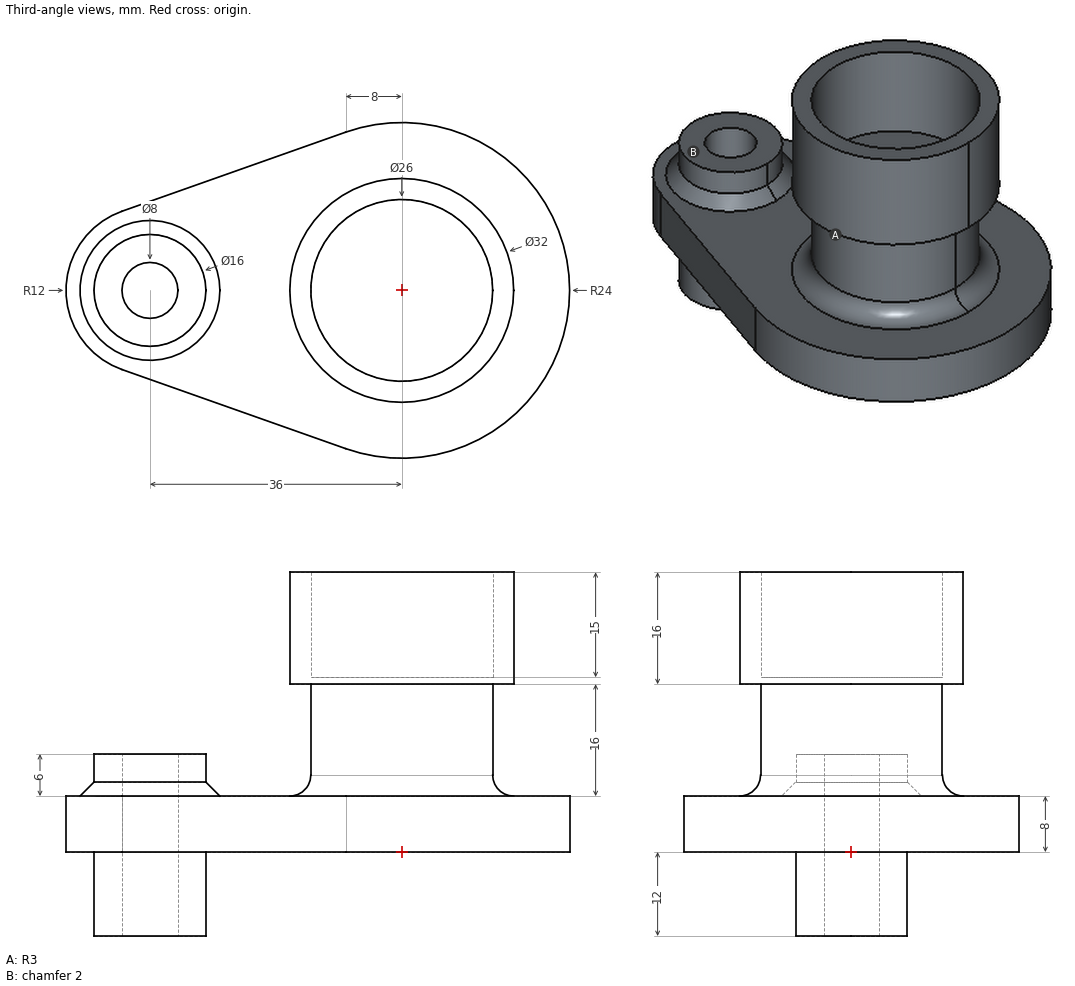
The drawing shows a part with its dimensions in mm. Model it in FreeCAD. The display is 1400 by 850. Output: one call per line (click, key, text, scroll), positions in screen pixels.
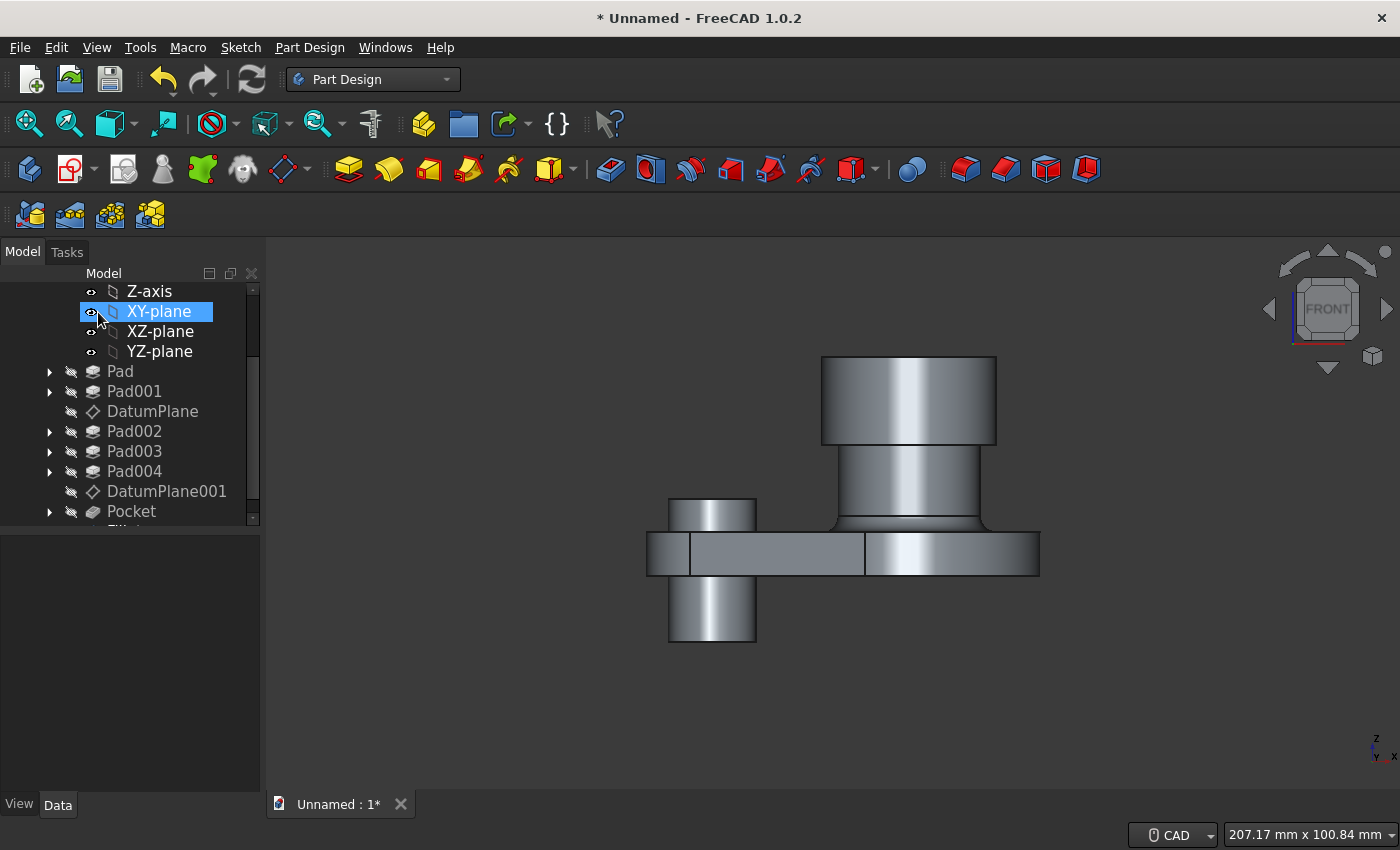
key(3)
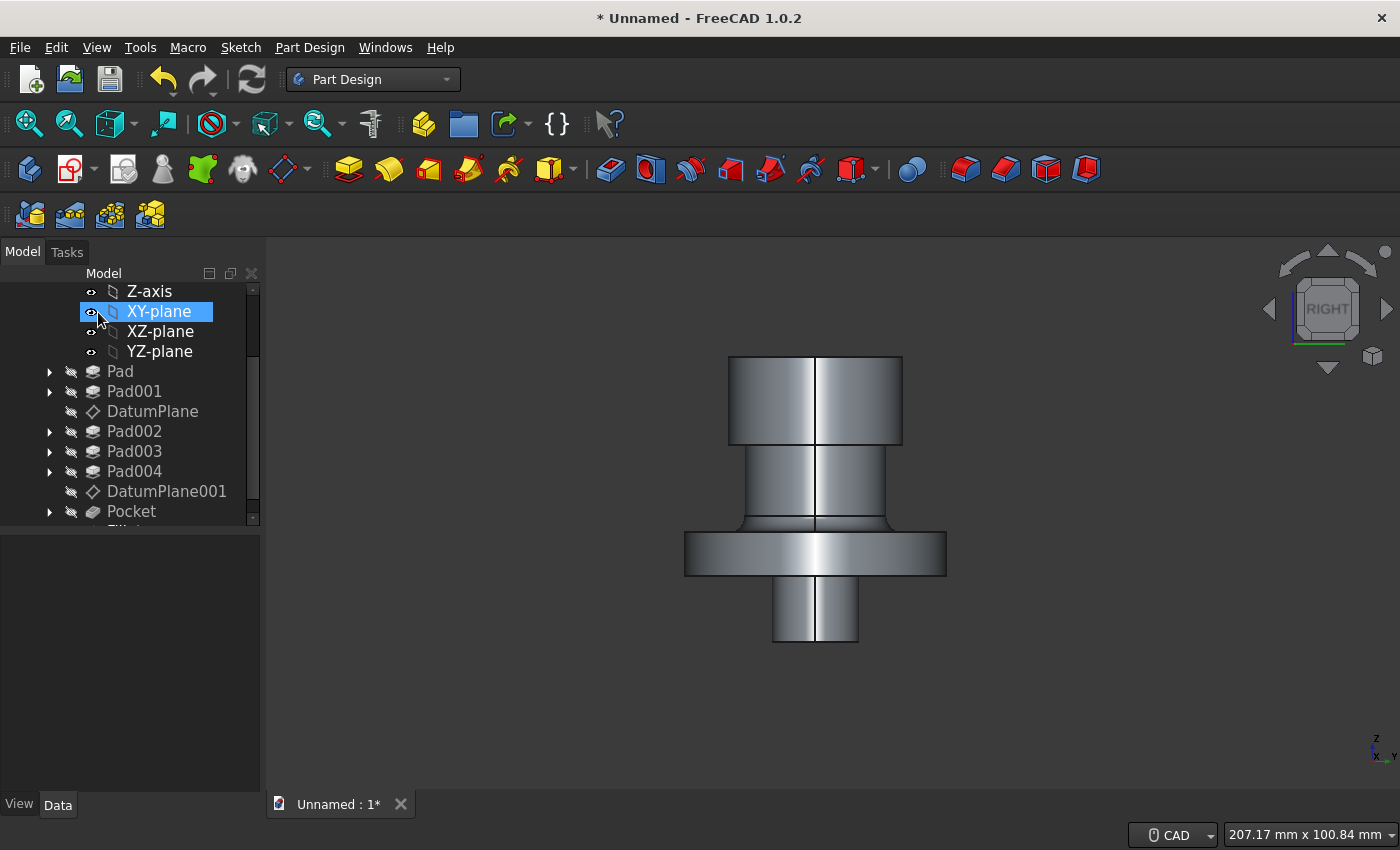
key(5)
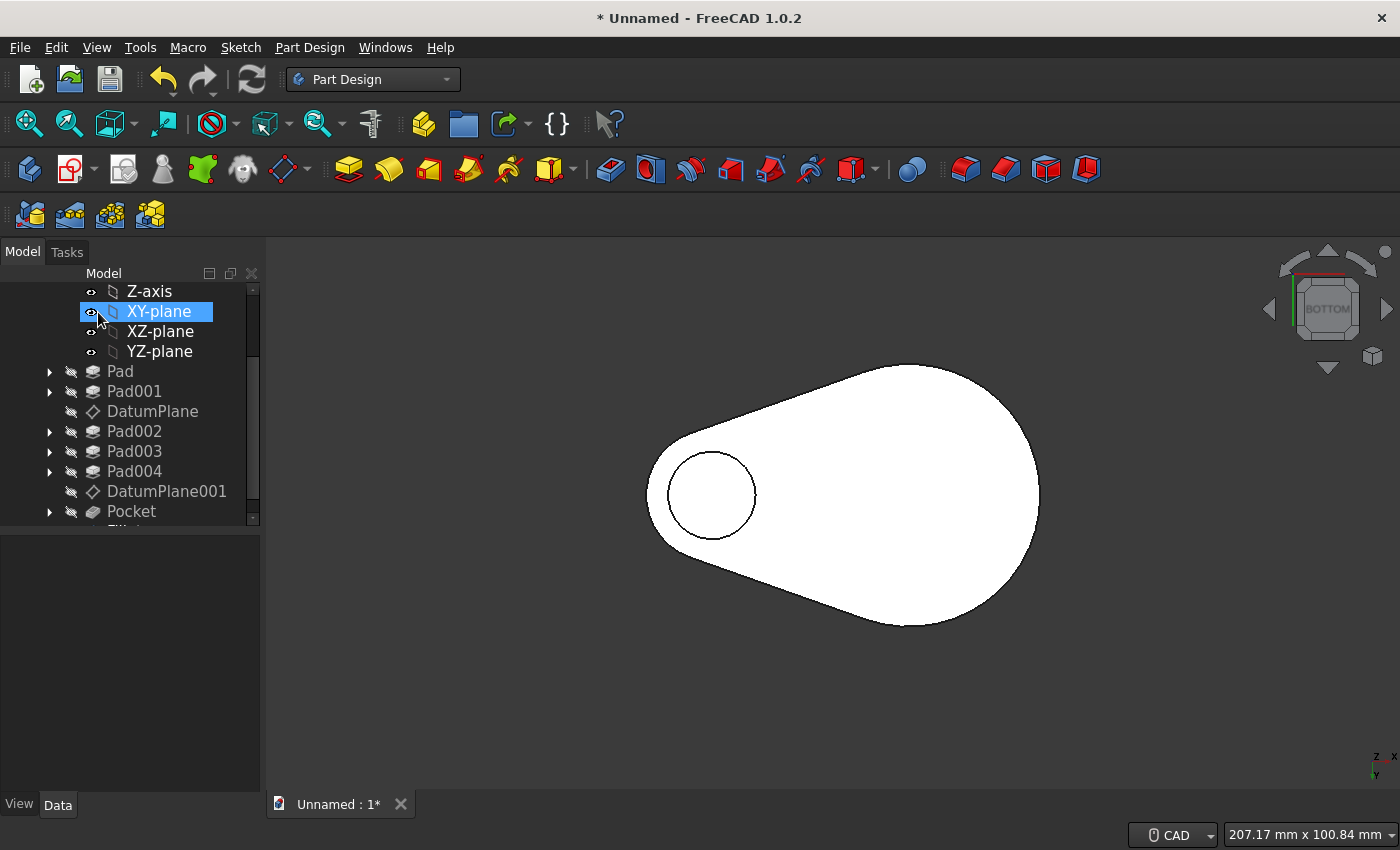
key(4)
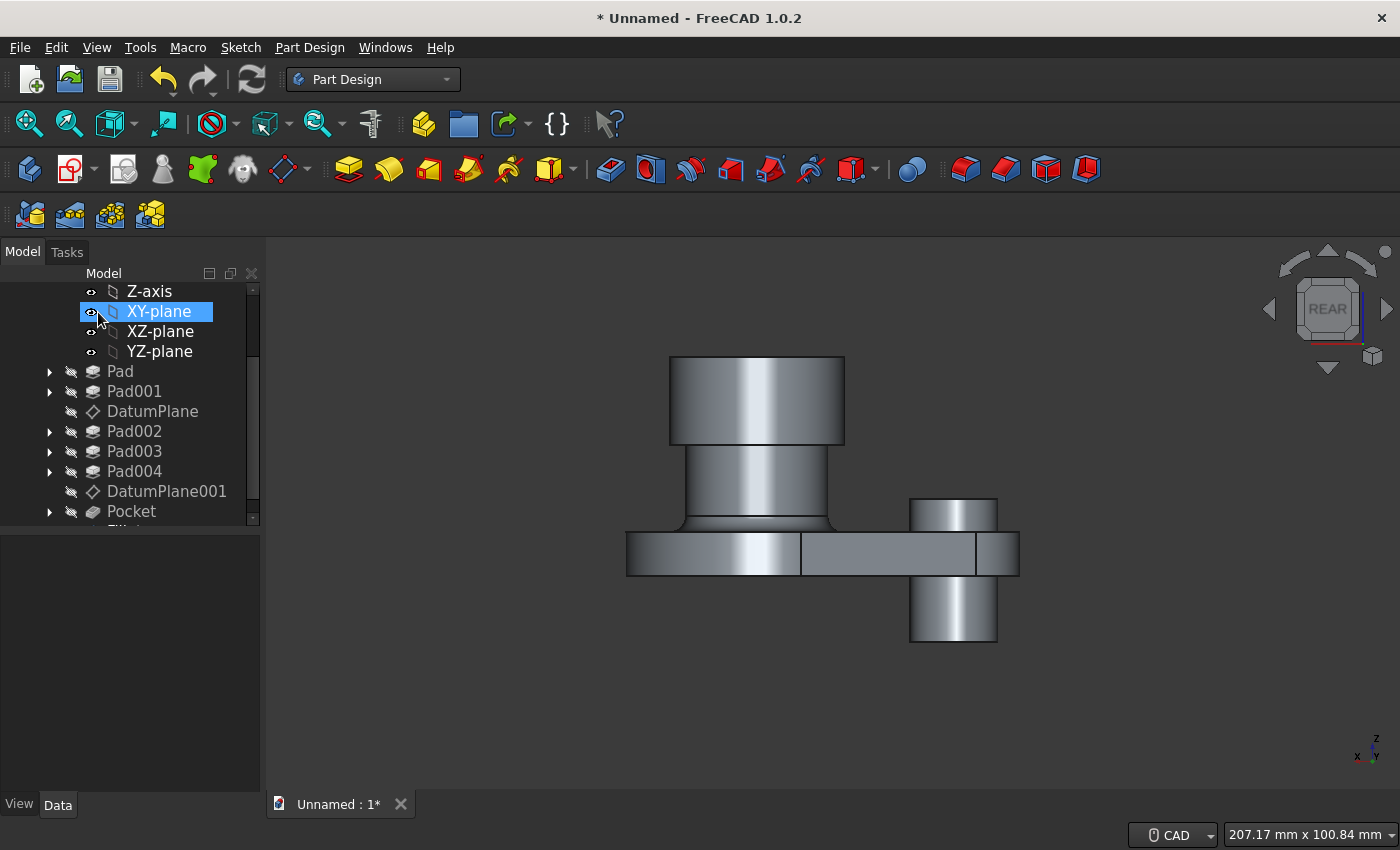
key(6)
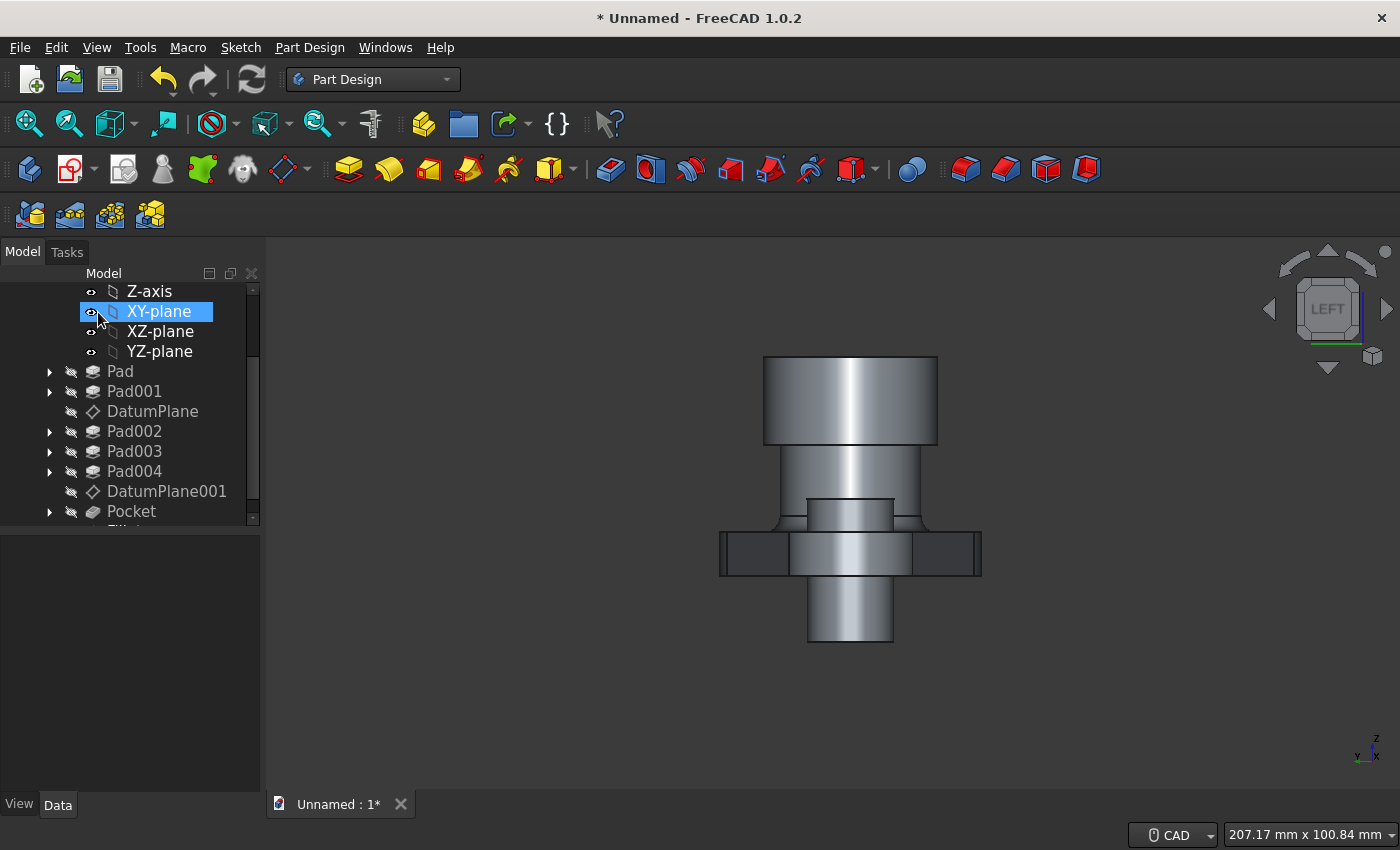
key(v)
key(3)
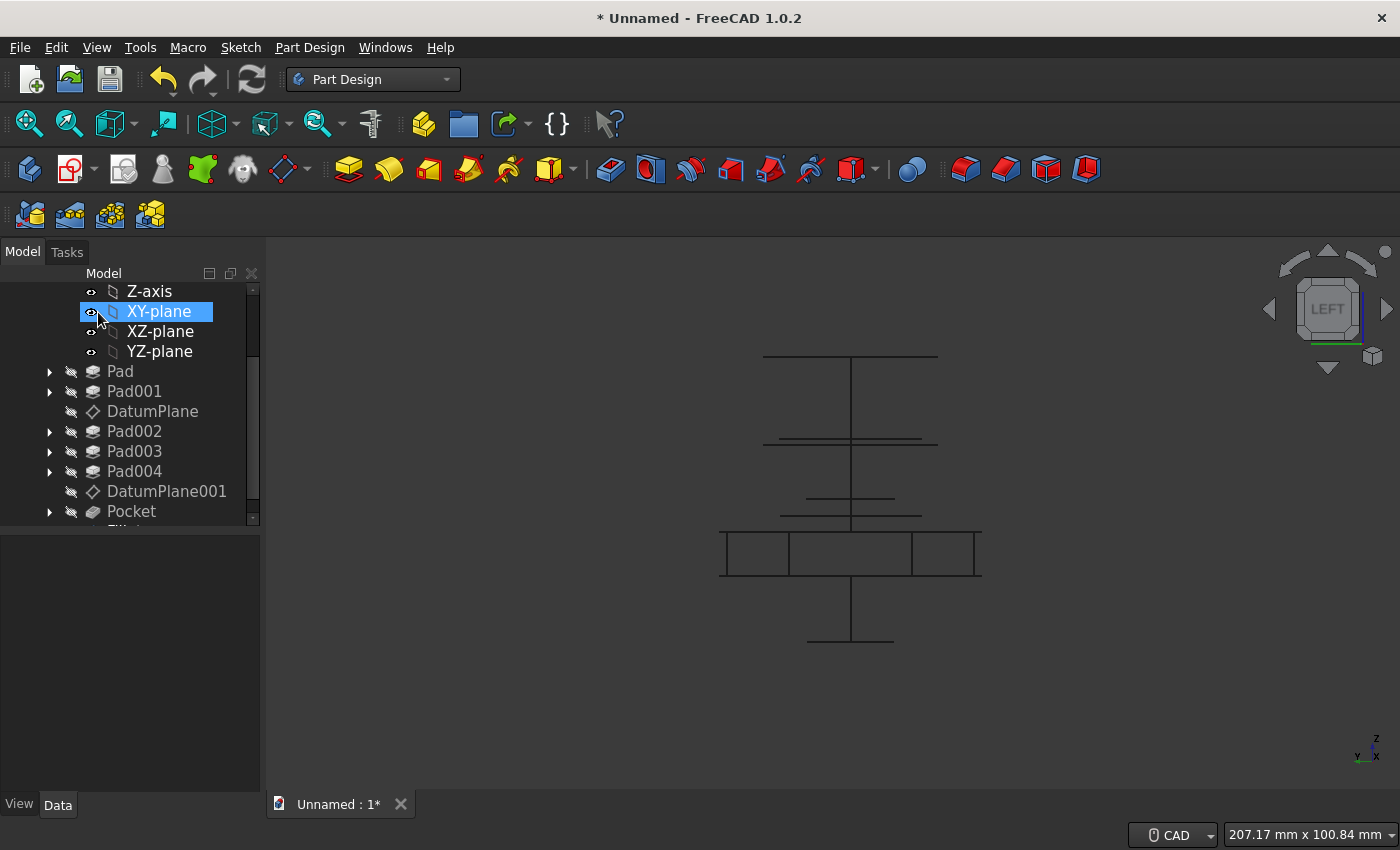
key(0)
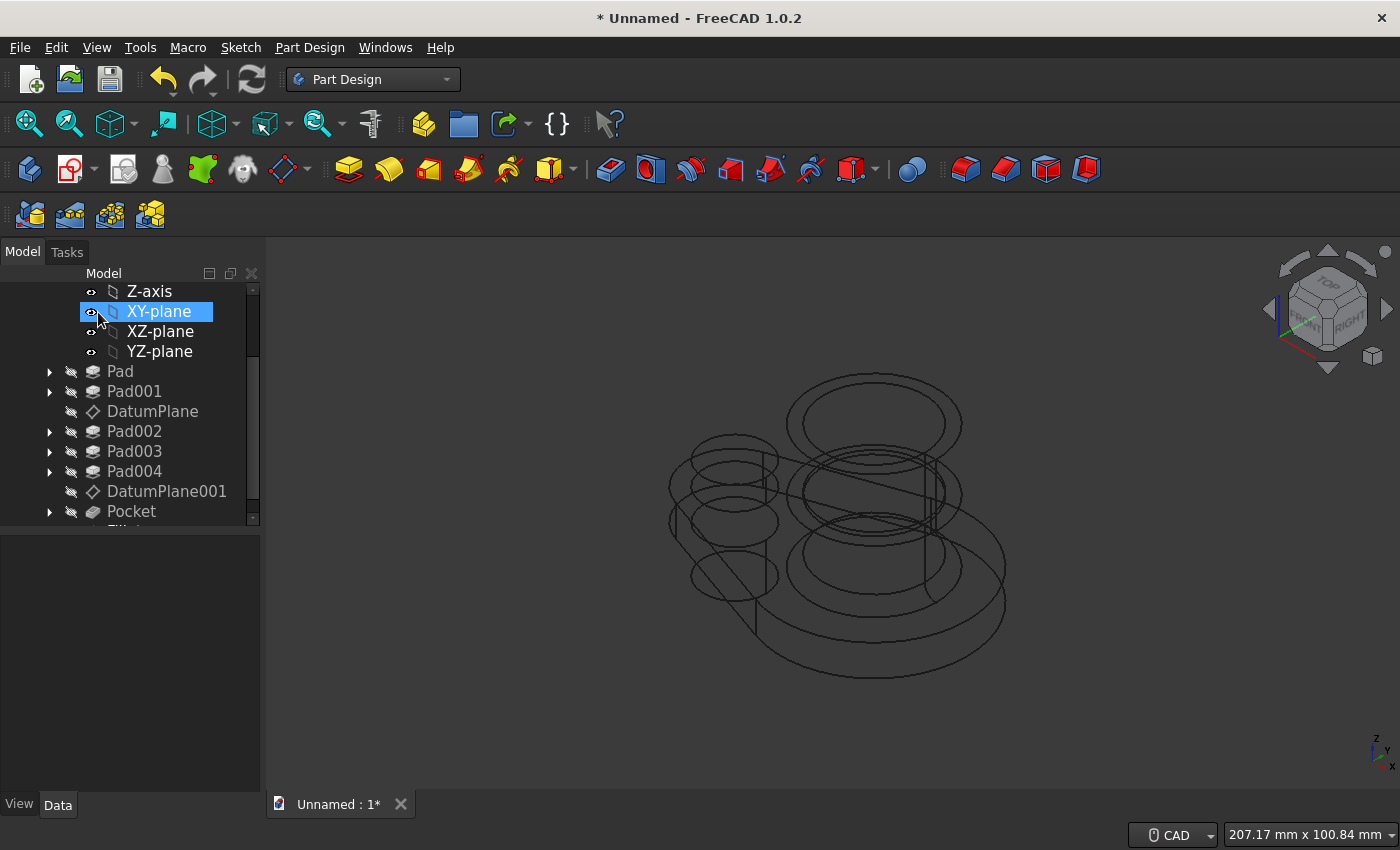
click(704, 468)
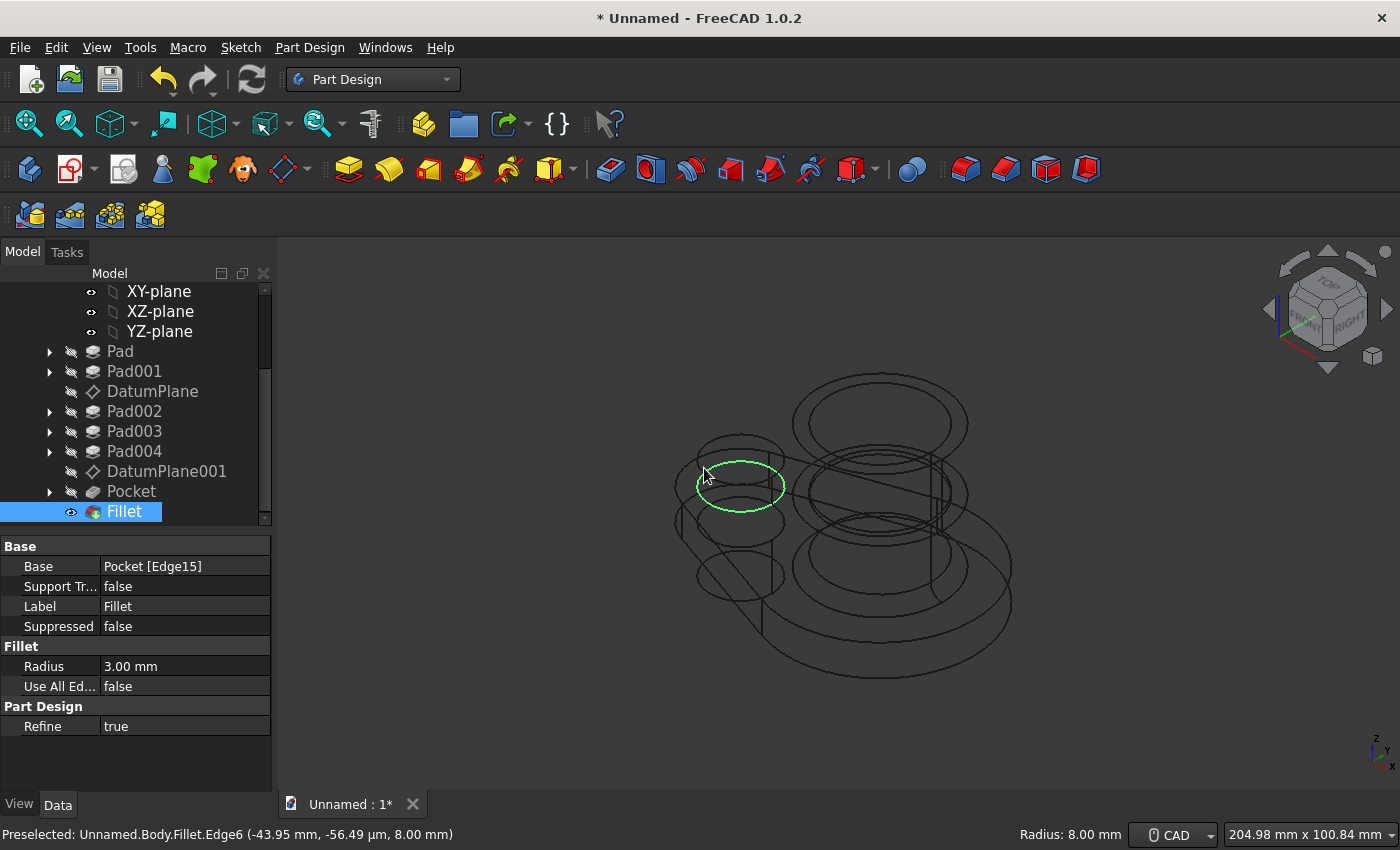
key(v)
key(1)